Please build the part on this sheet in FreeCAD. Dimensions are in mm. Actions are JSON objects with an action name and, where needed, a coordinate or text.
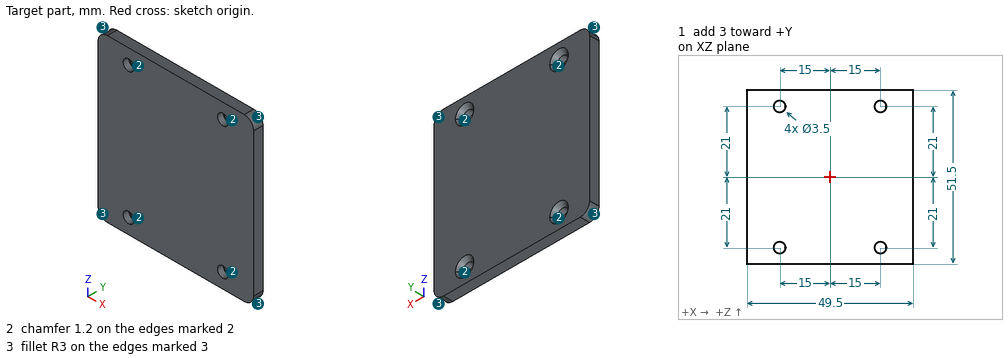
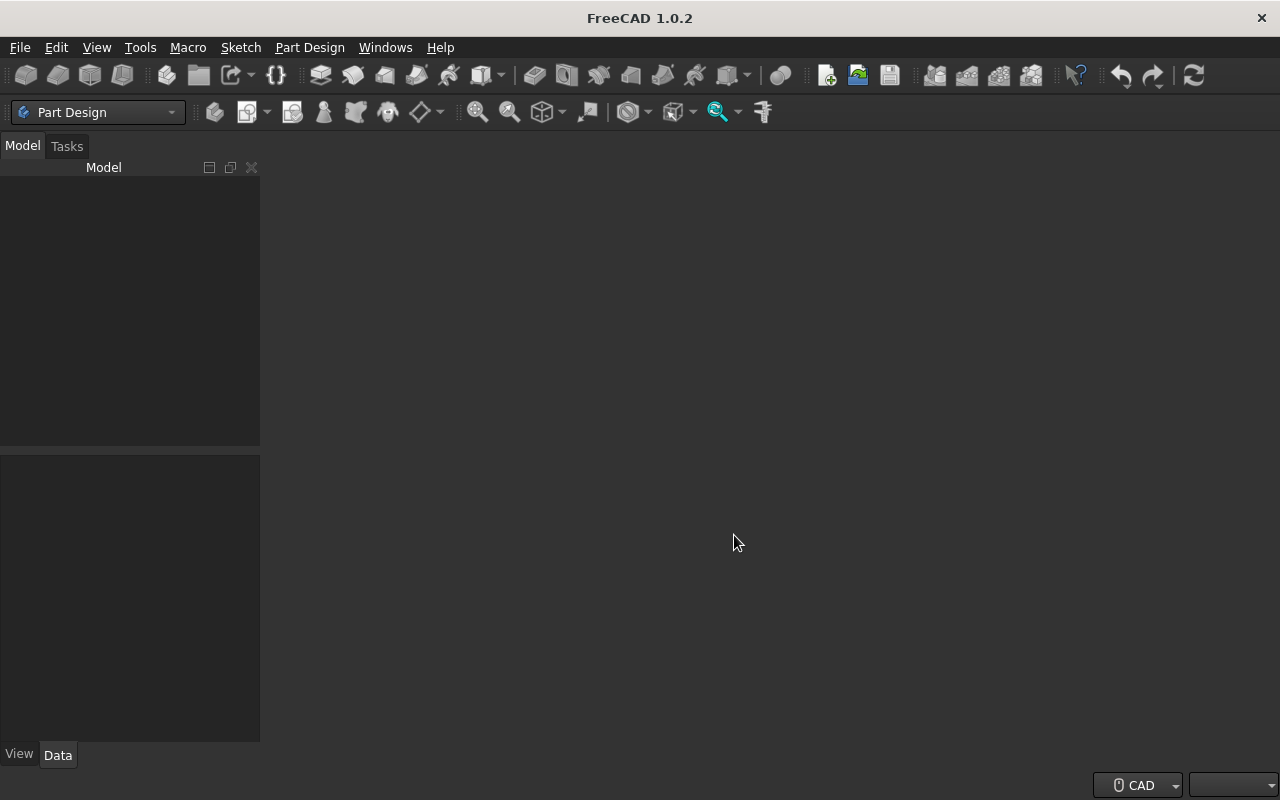
{"action": "left_click", "coordinate": [826, 76]}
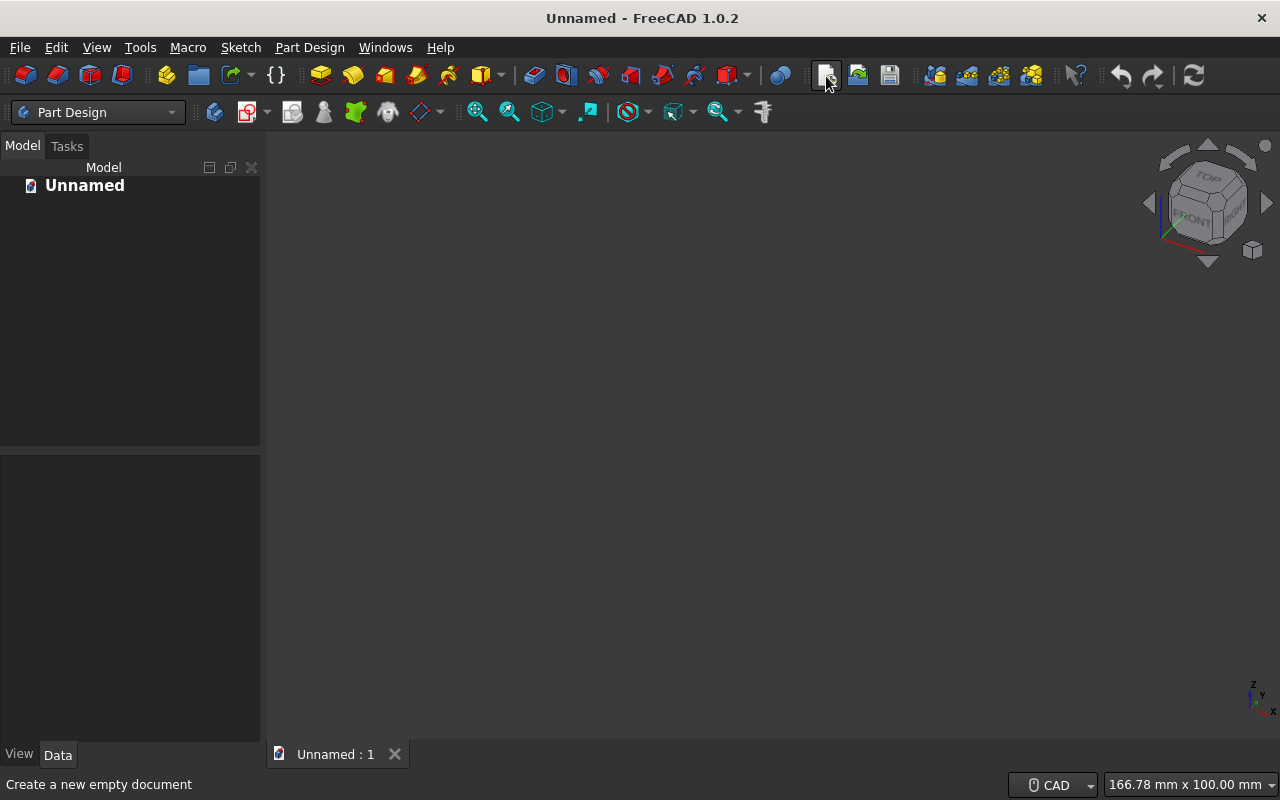
{"action": "left_click", "coordinate": [248, 112]}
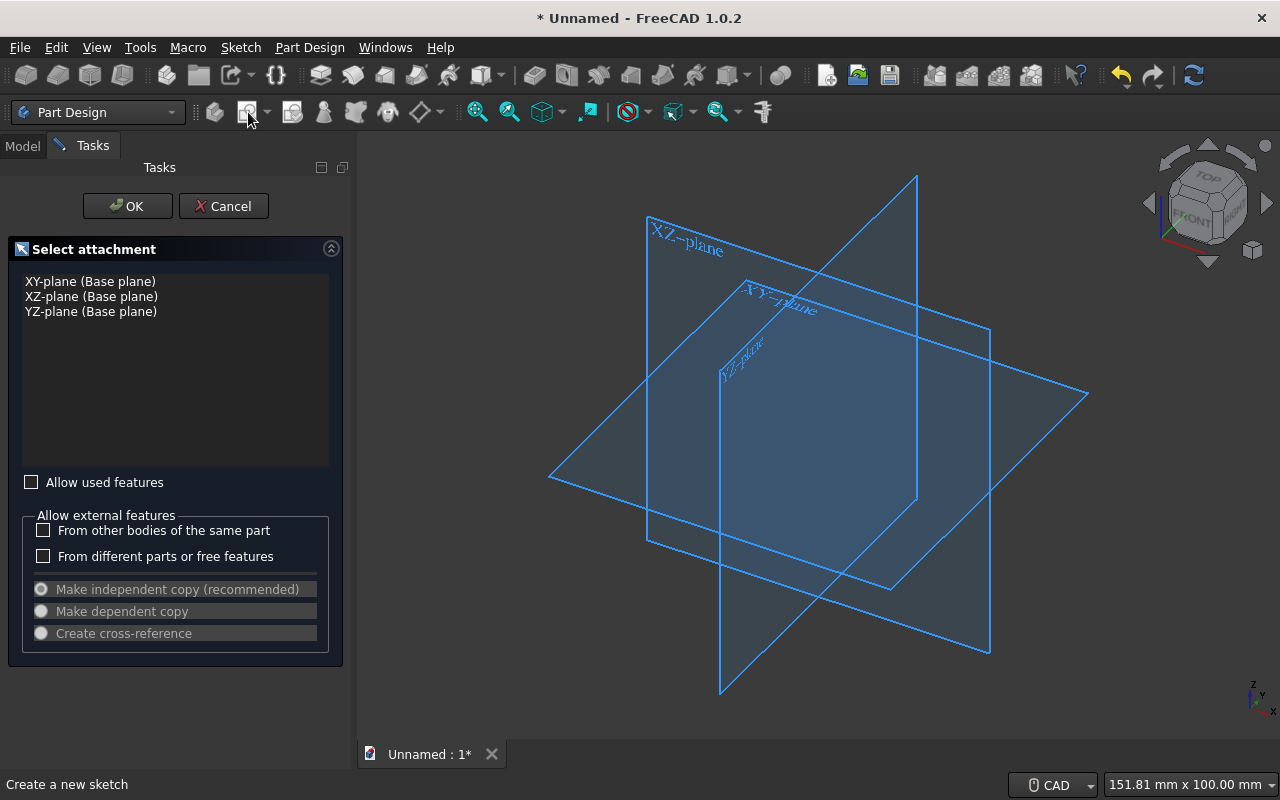
{"action": "left_click", "coordinate": [82, 296]}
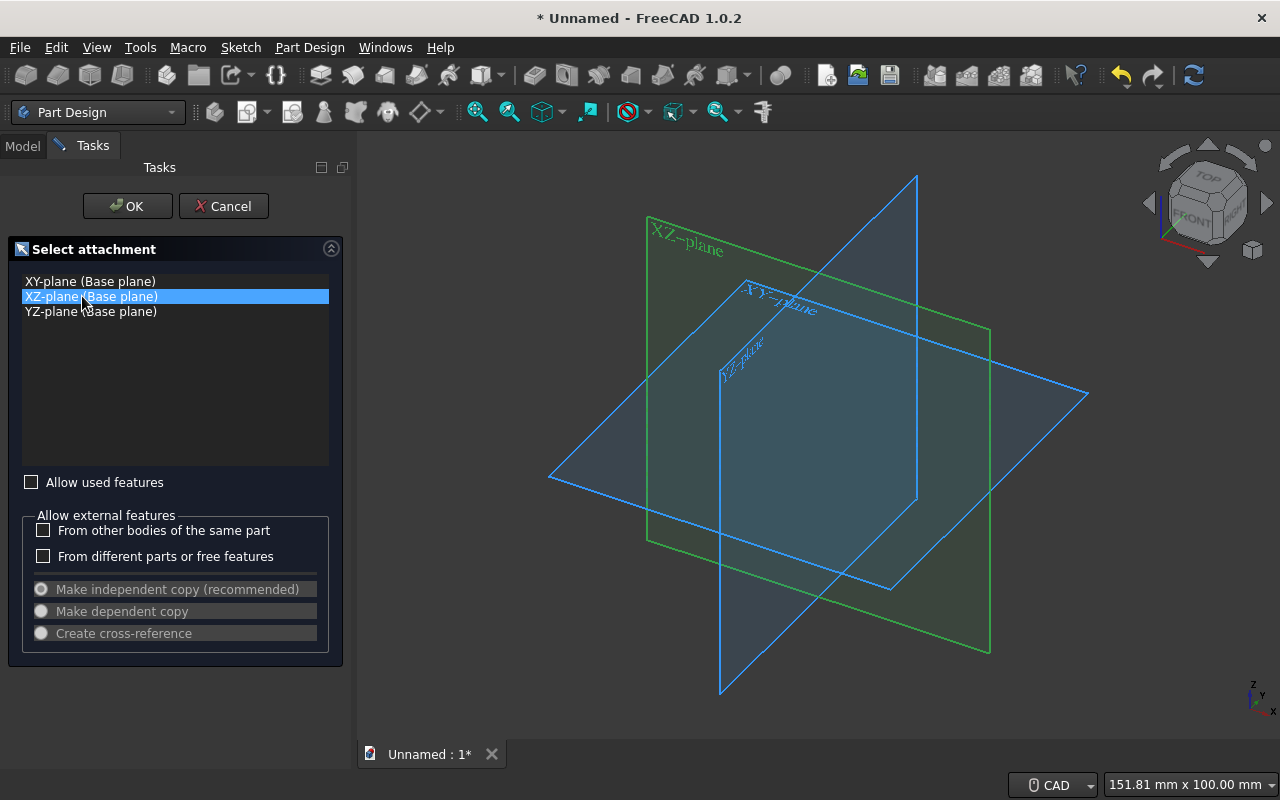
{"action": "left_click", "coordinate": [128, 206]}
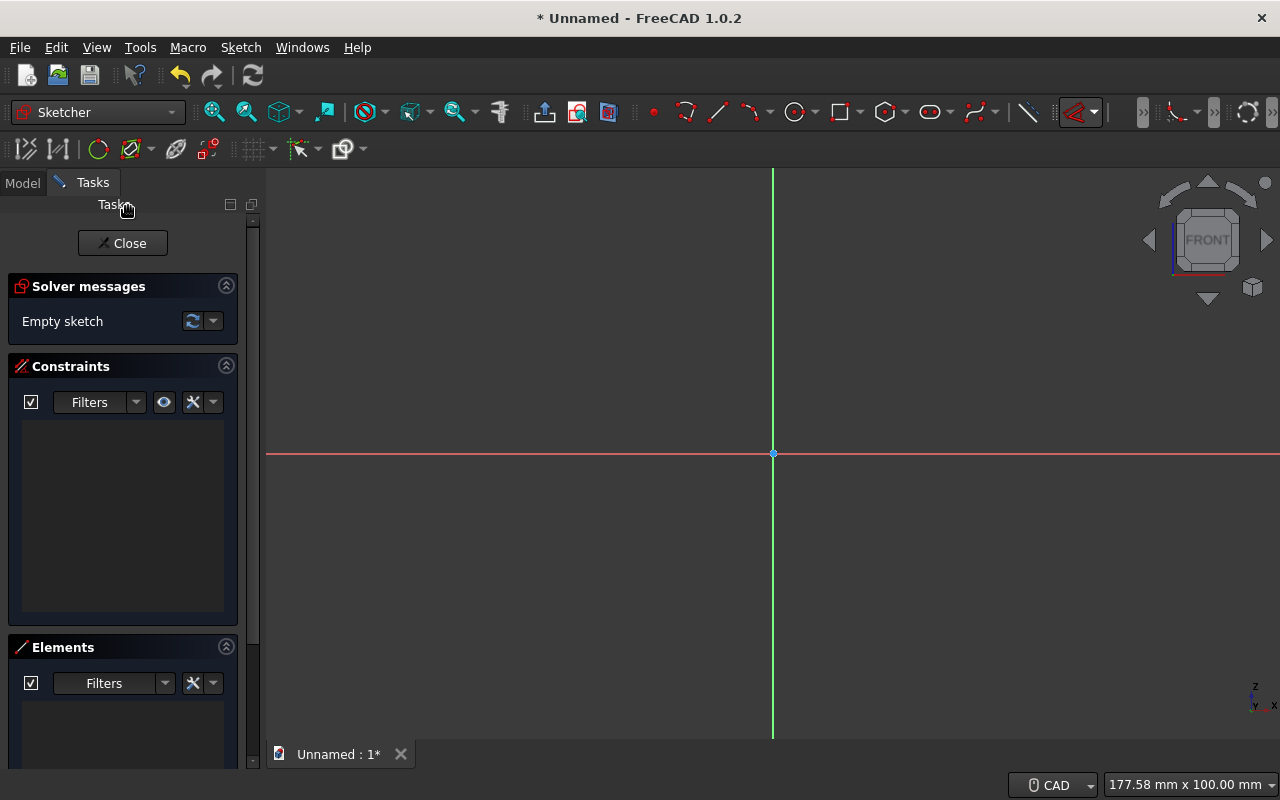
{"action": "left_click", "coordinate": [862, 112]}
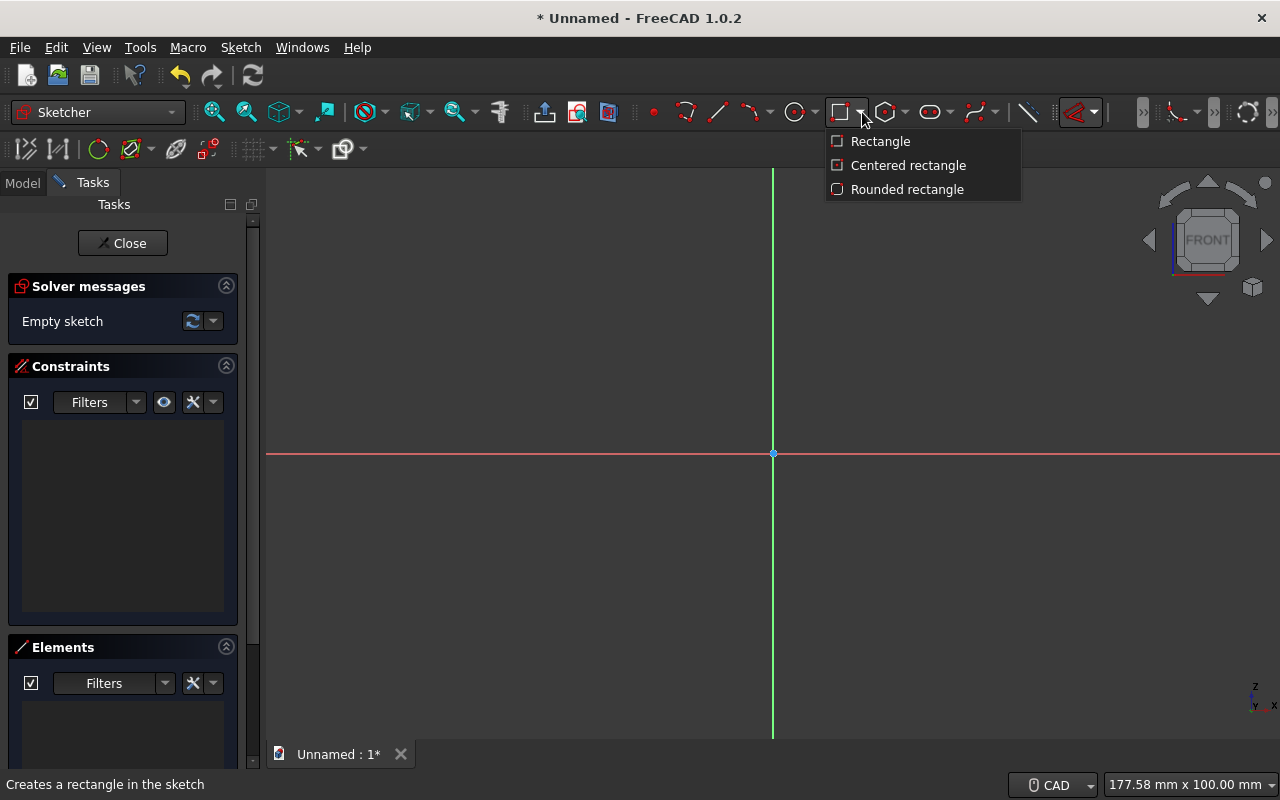
{"action": "left_click", "coordinate": [924, 165]}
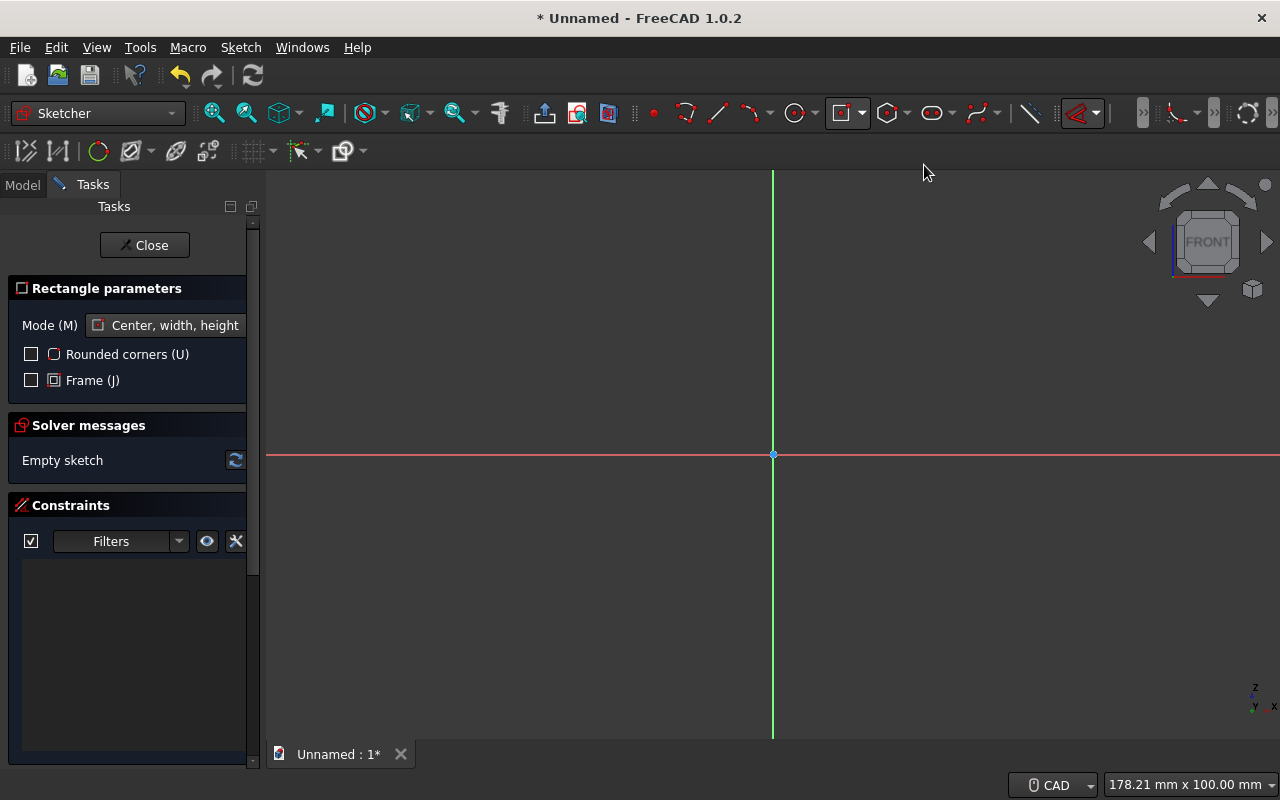
{"action": "left_click", "coordinate": [773, 454]}
{"action": "left_click", "coordinate": [914, 308]}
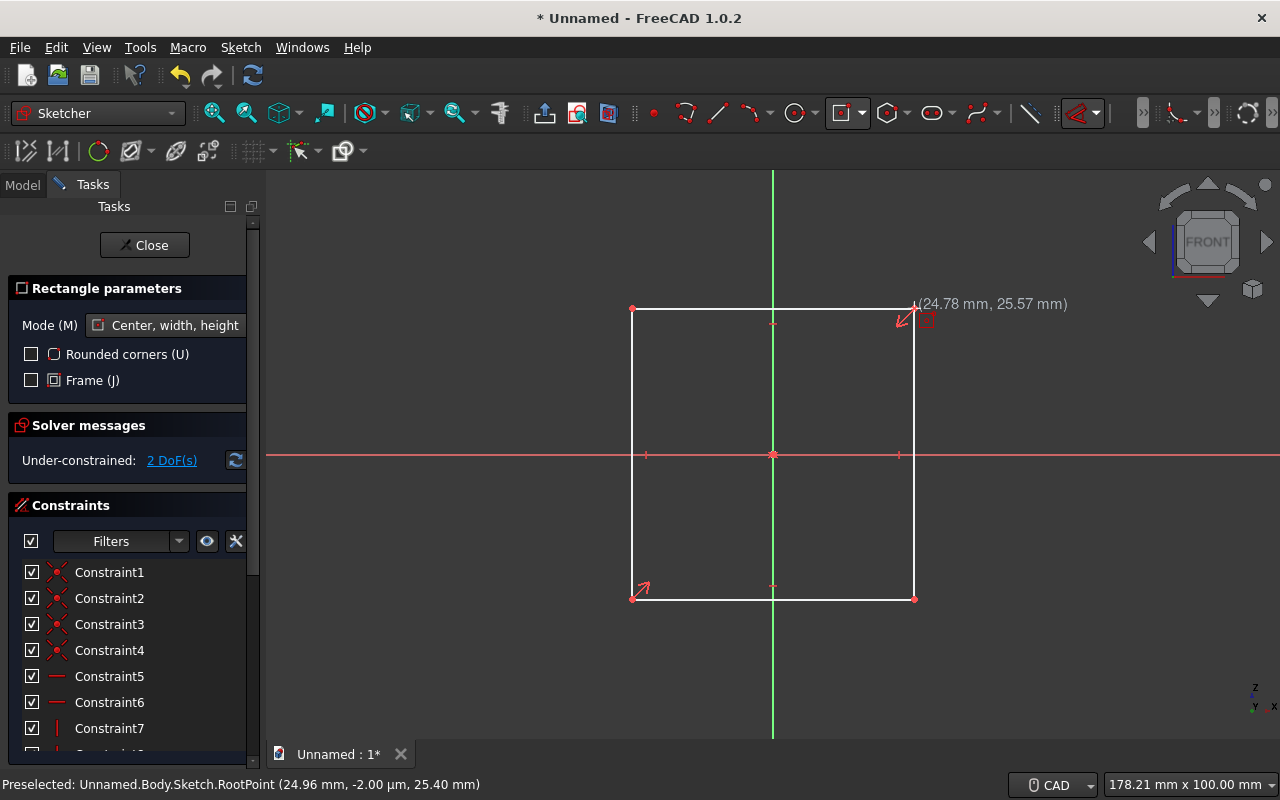
{"action": "left_click", "coordinate": [796, 114]}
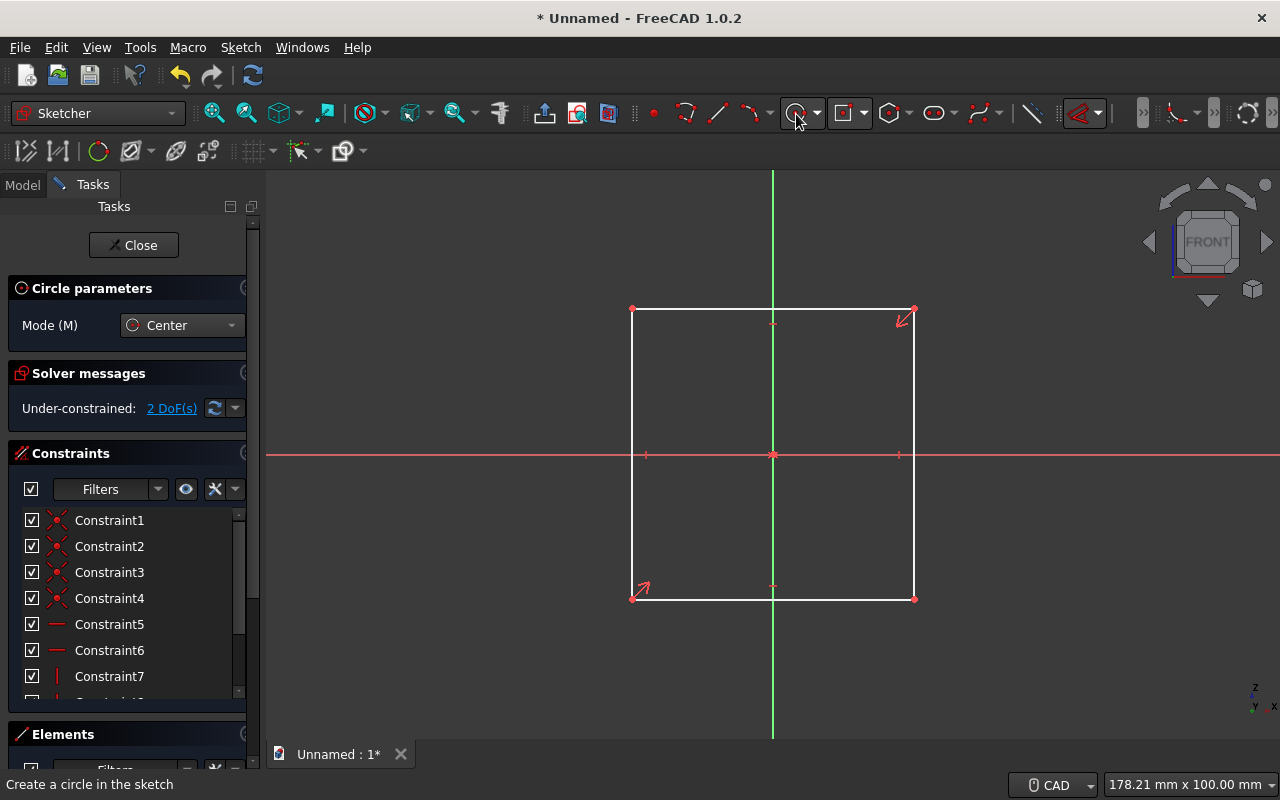
{"action": "scroll", "coordinate": [688, 335], "scroll_direction": "up", "scroll_amount": 5}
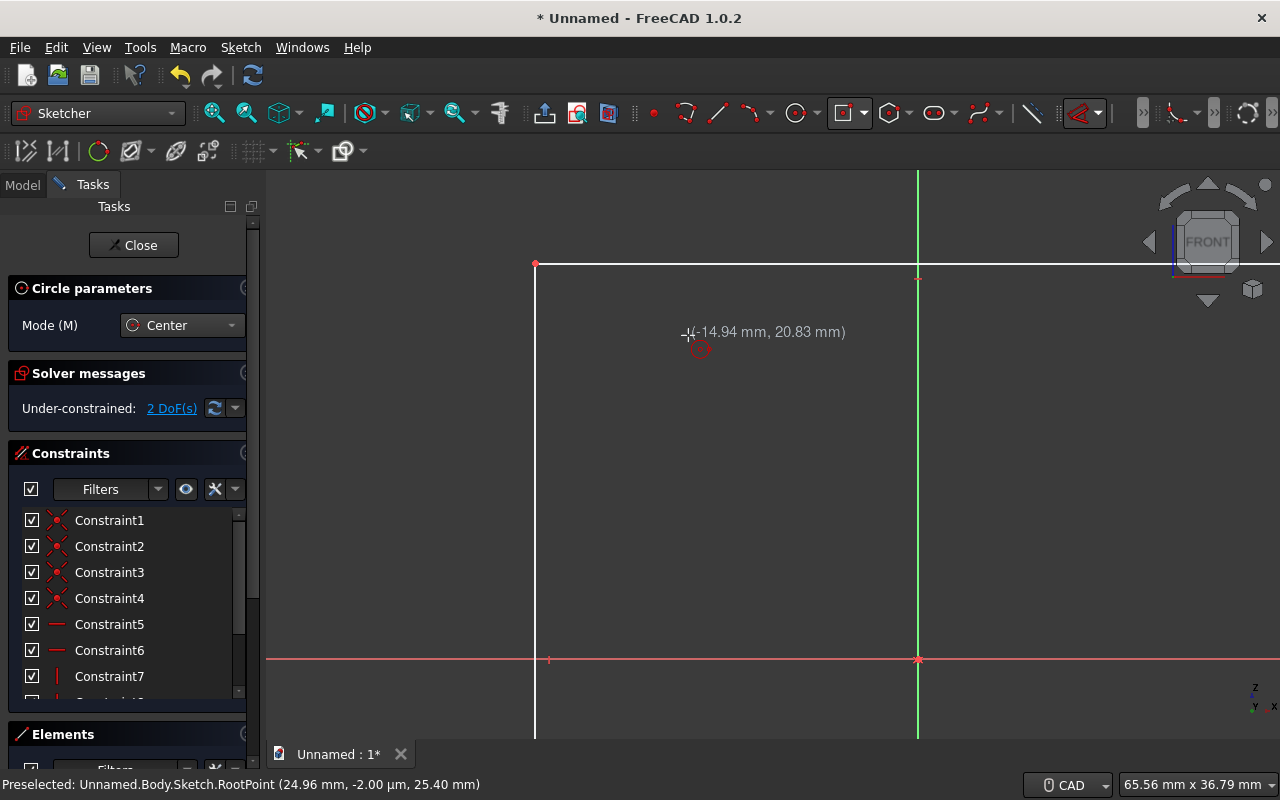
{"action": "left_click", "coordinate": [686, 335]}
{"action": "left_click", "coordinate": [705, 315]}